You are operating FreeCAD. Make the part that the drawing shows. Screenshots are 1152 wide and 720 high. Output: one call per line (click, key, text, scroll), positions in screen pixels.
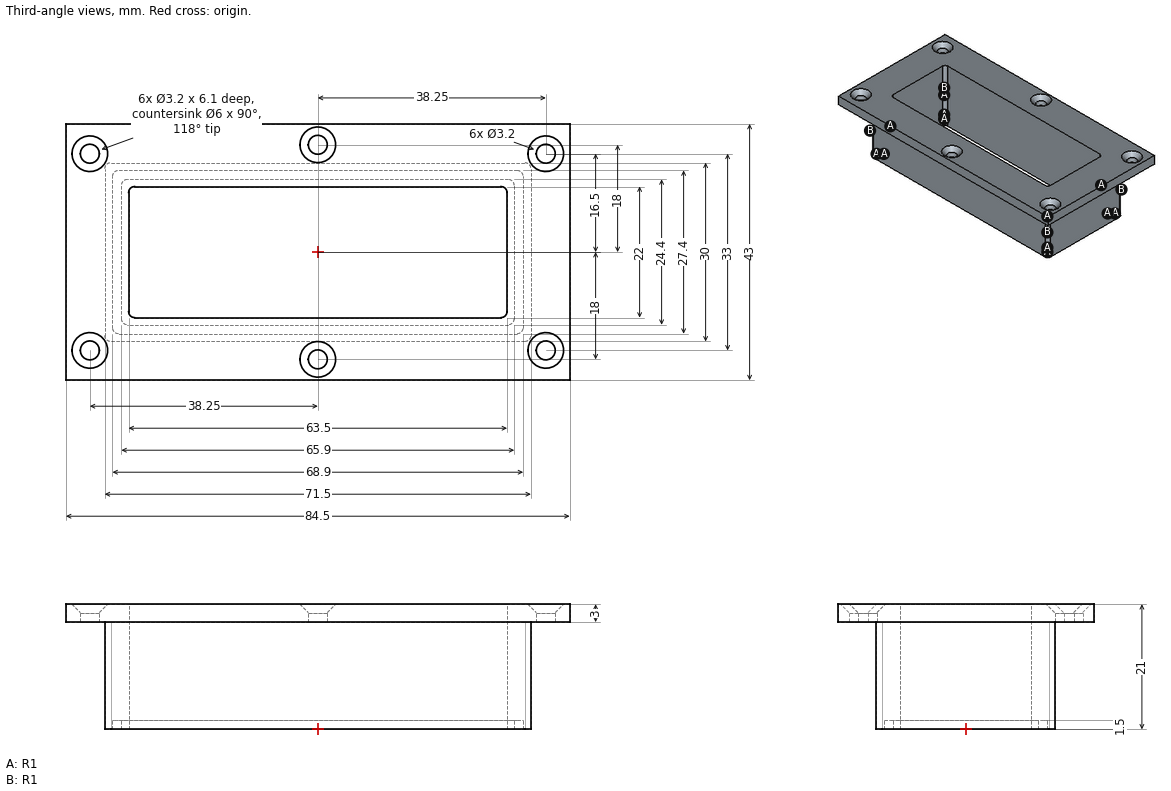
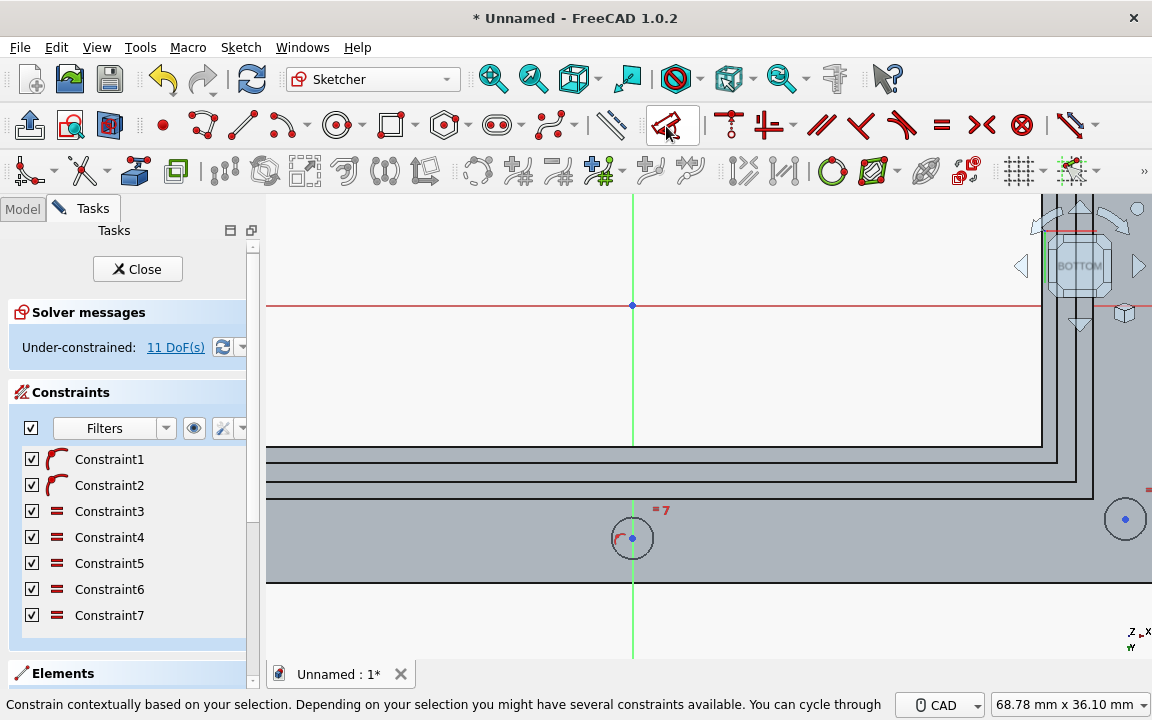
scroll(647, 525, down, 4)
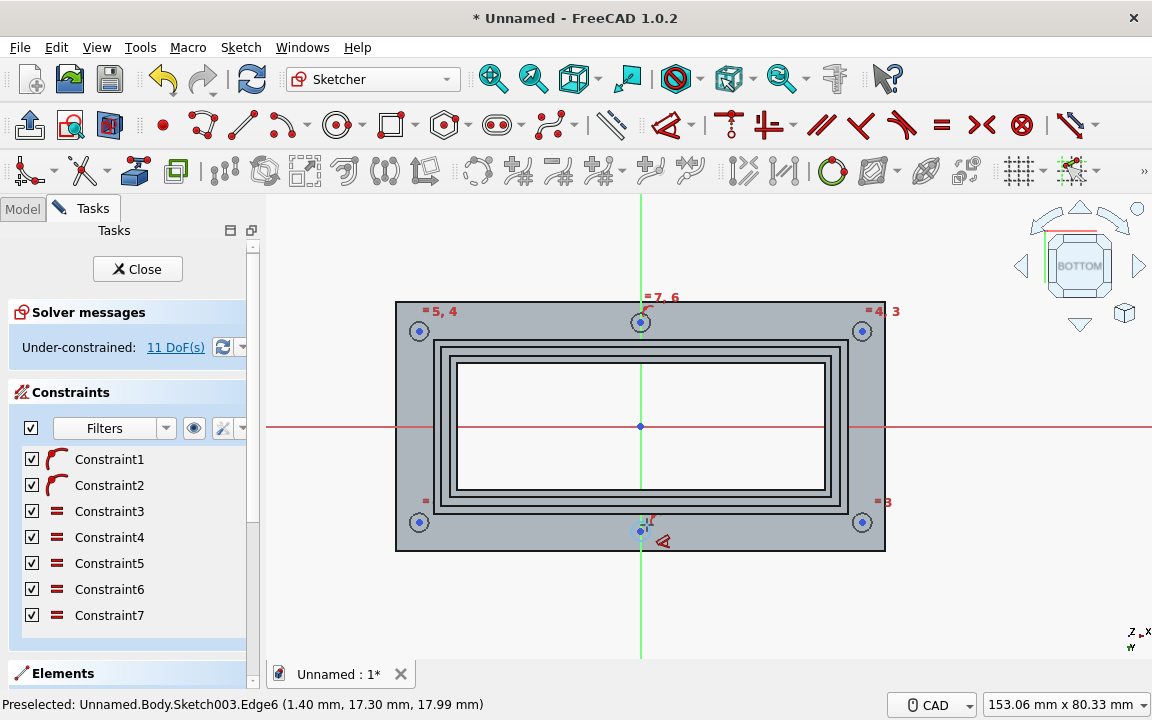
scroll(869, 516, up, 4)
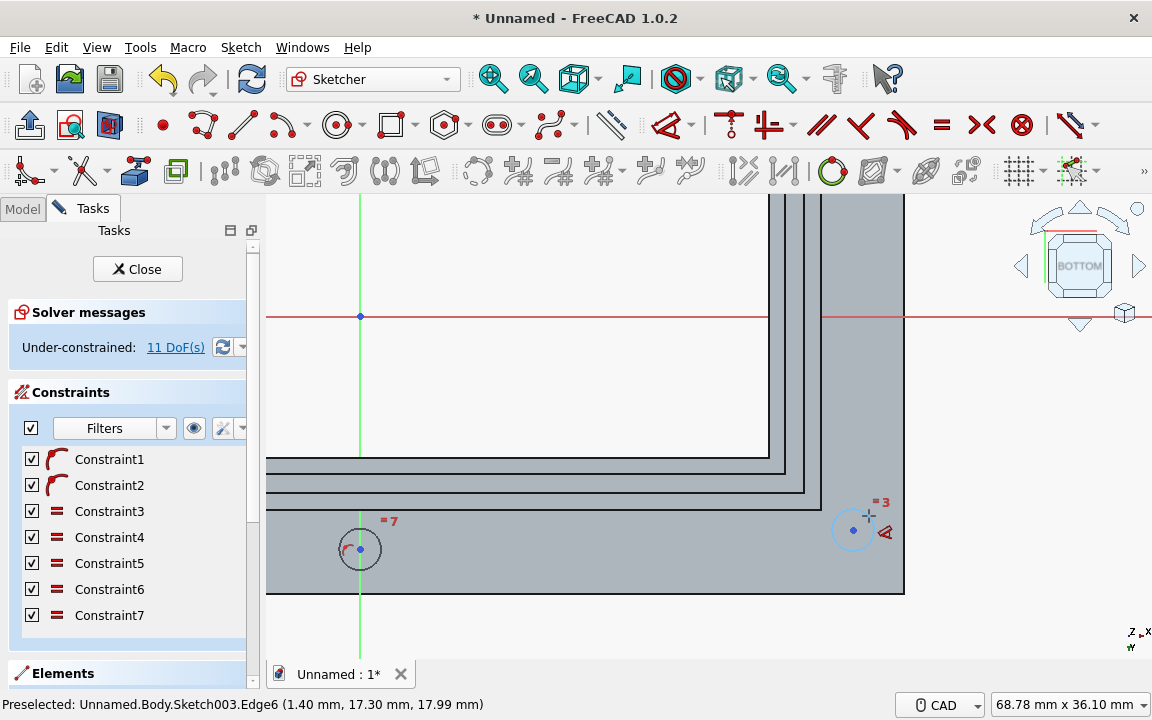
click(868, 515)
click(890, 492)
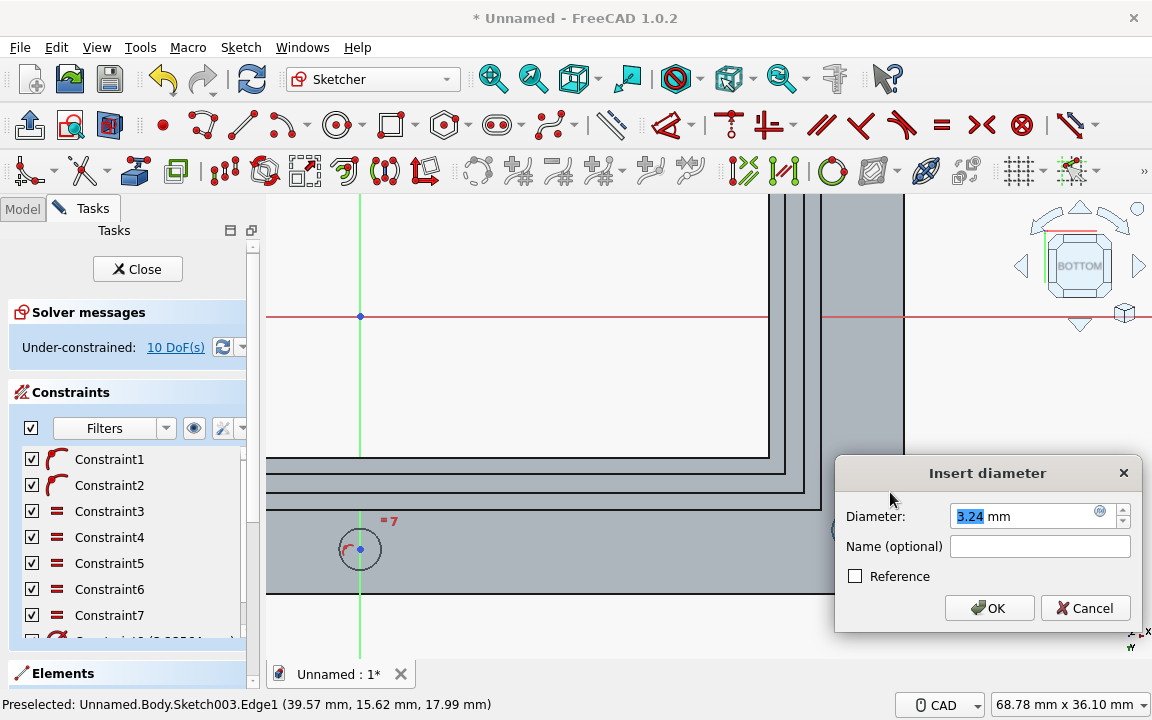
text(3.2)
key(Return)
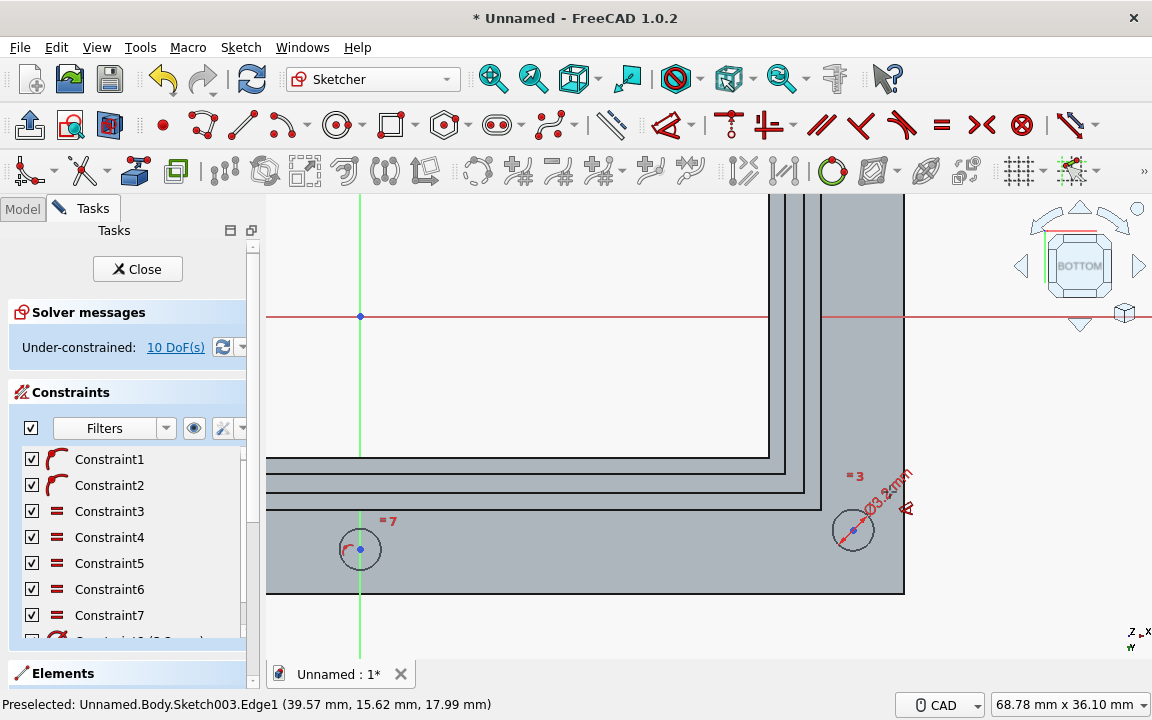
scroll(869, 516, down, 4)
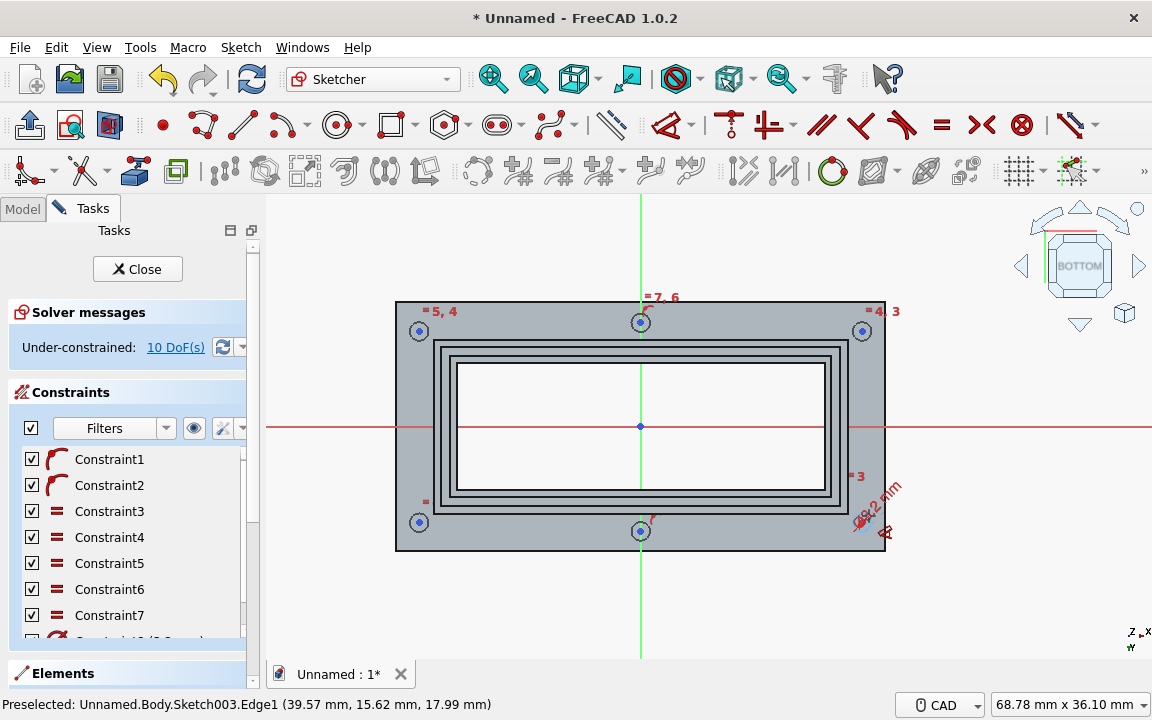
click(641, 323)
click(675, 375)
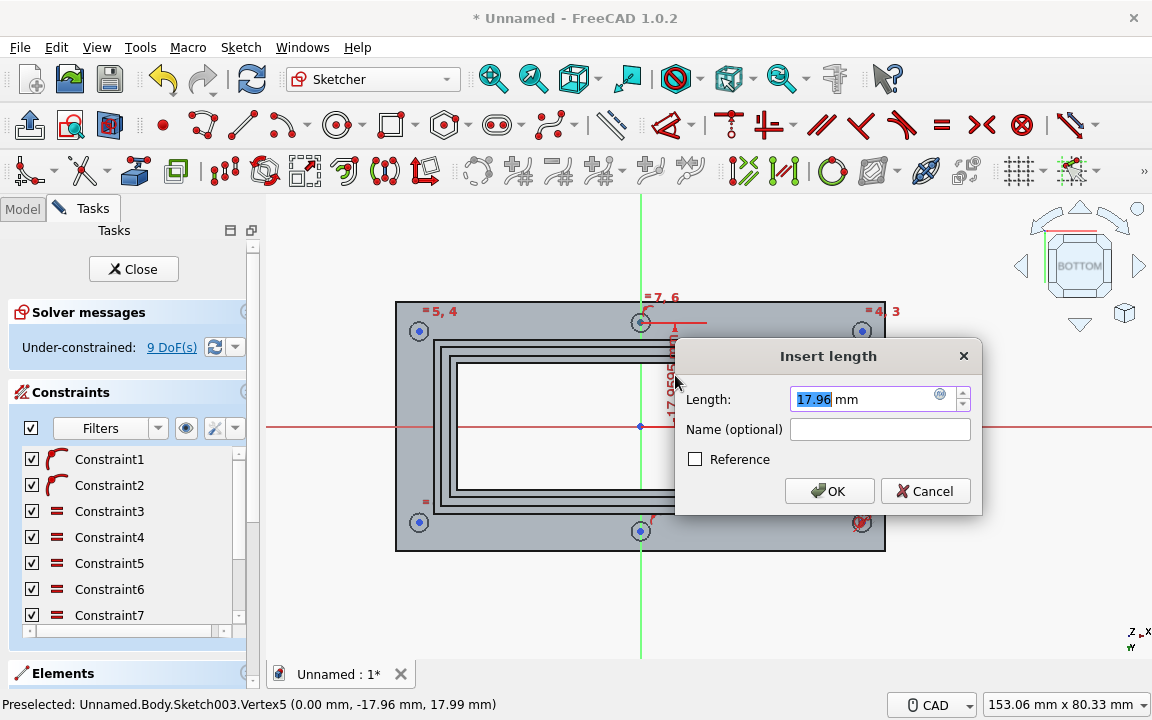
text(18)
key(Return)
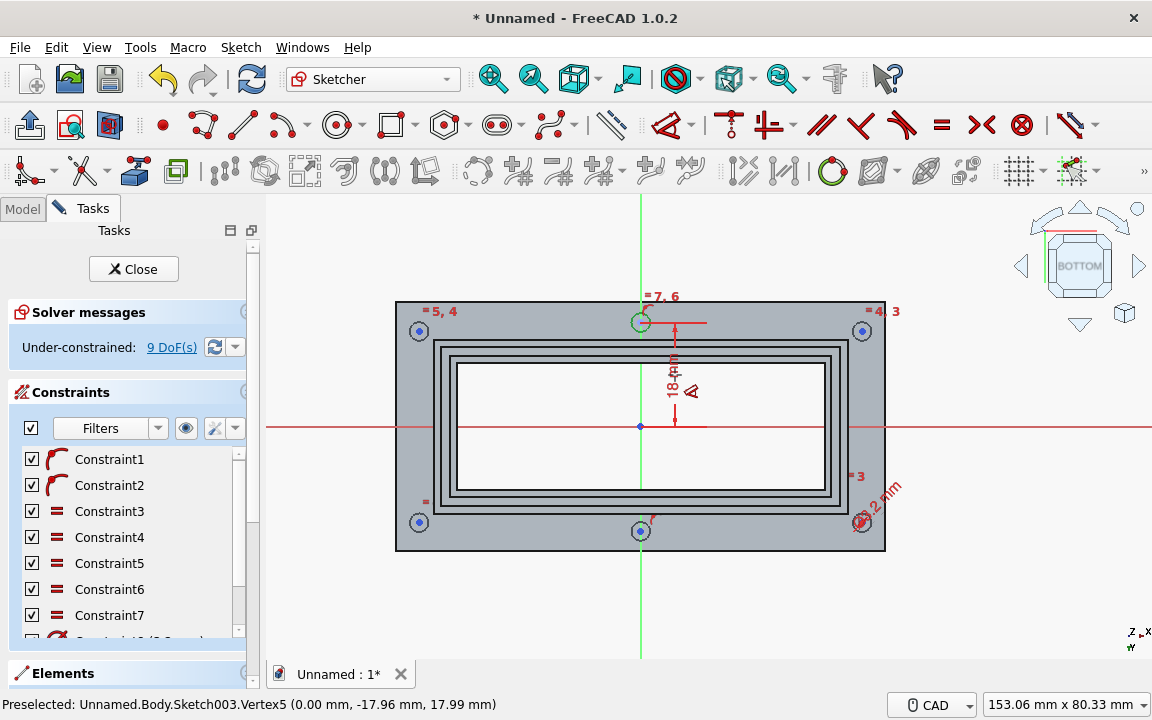
click(641, 531)
click(675, 479)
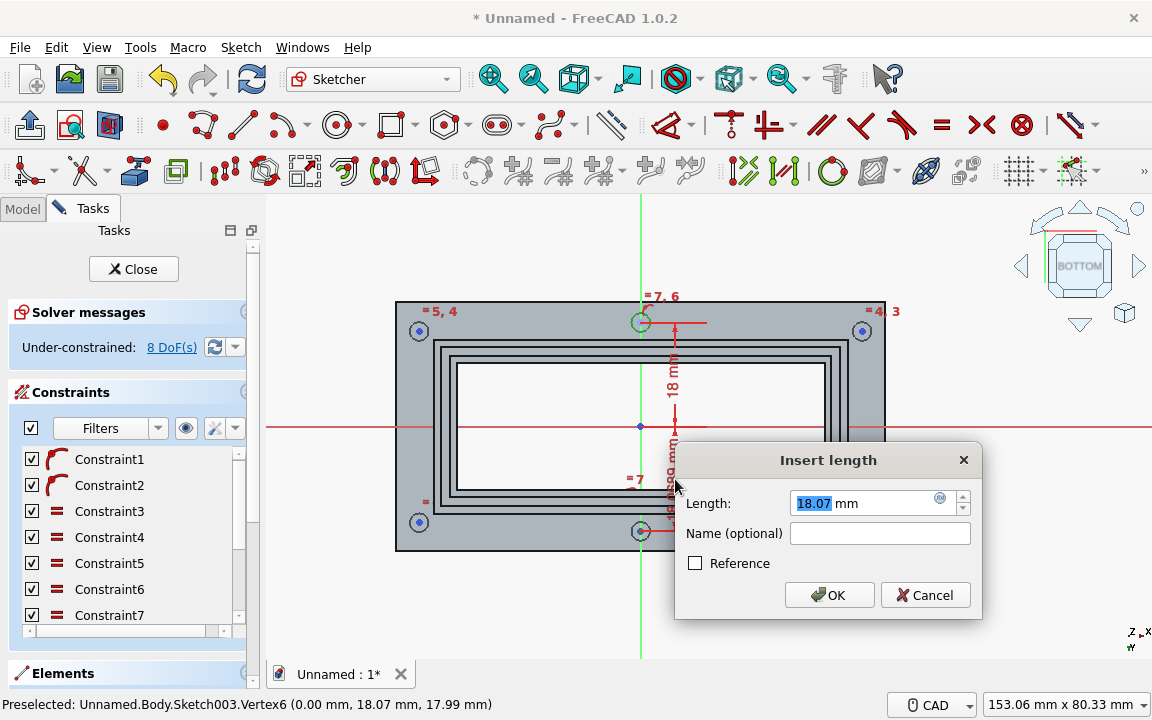
text(18)
key(Return)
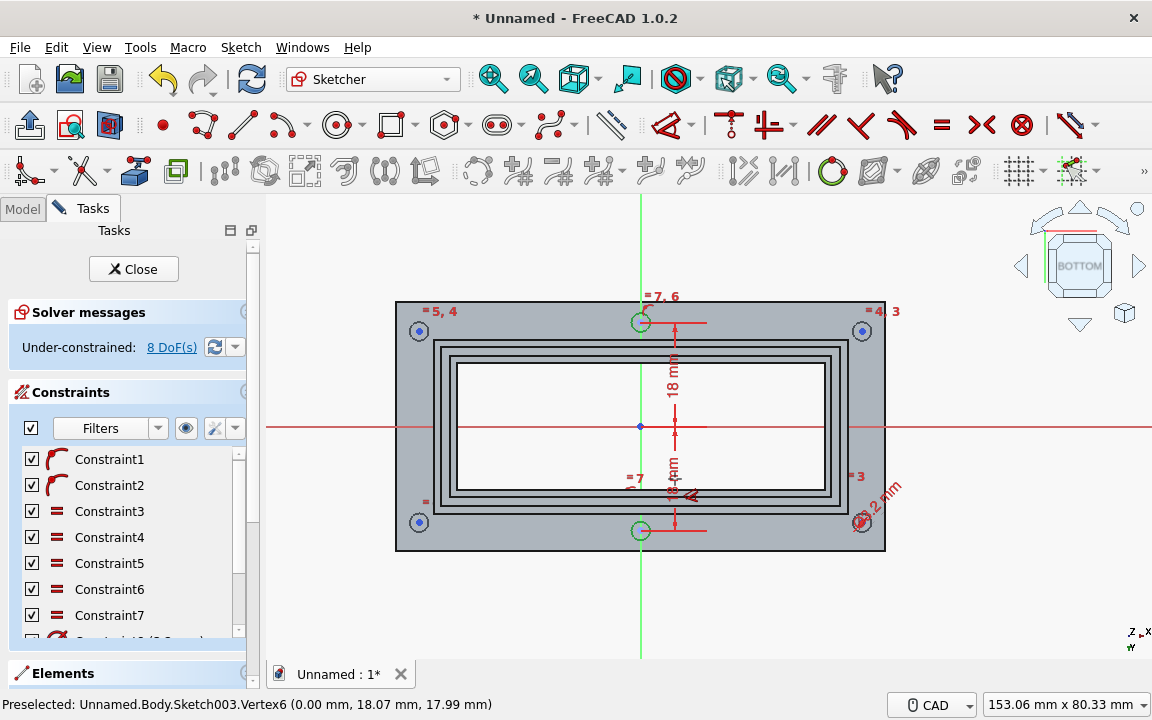
click(862, 523)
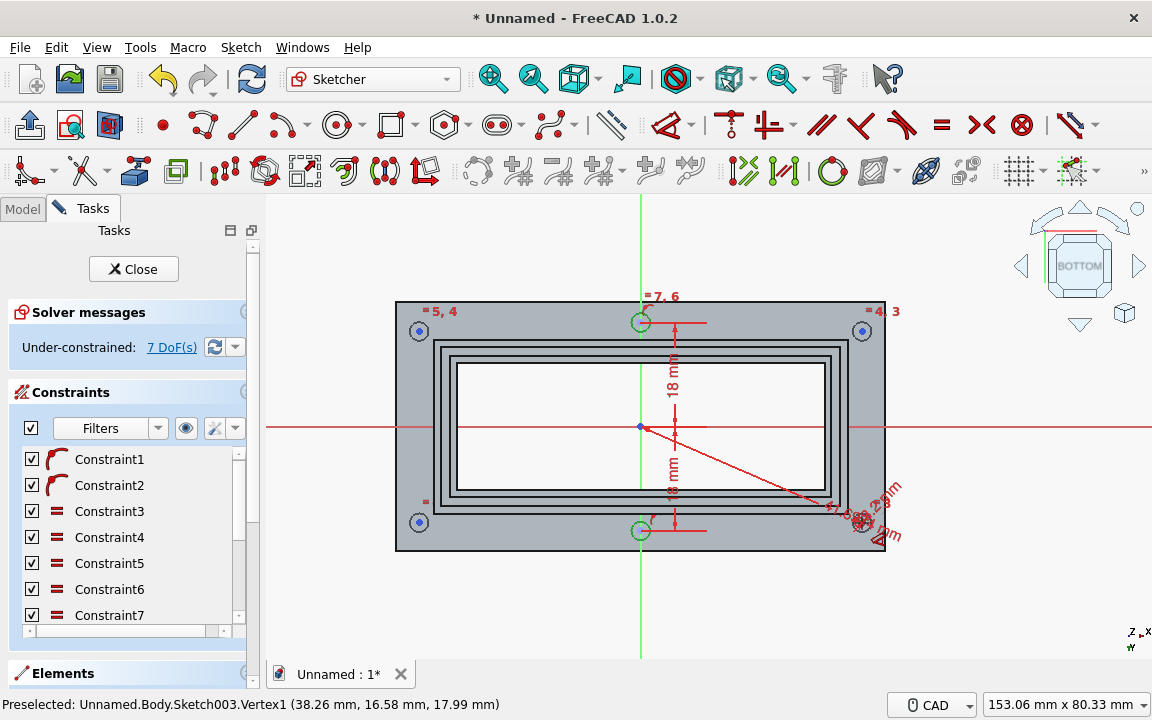
click(862, 331)
click(896, 383)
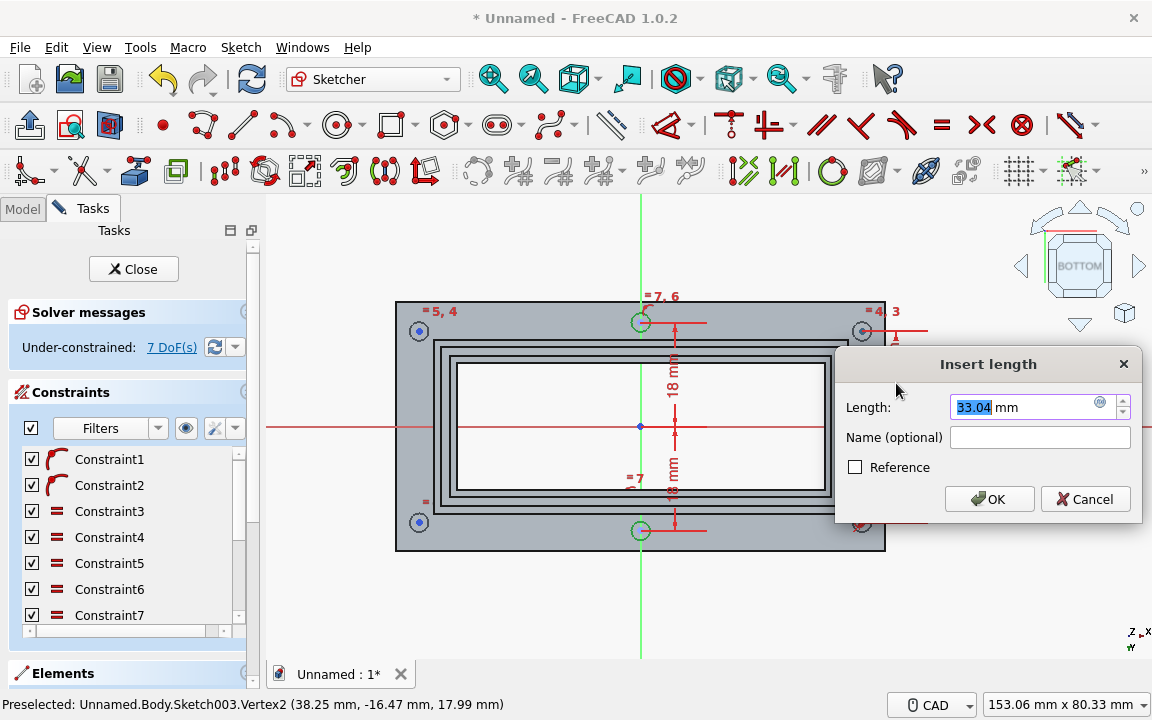
text(33)
key(Return)